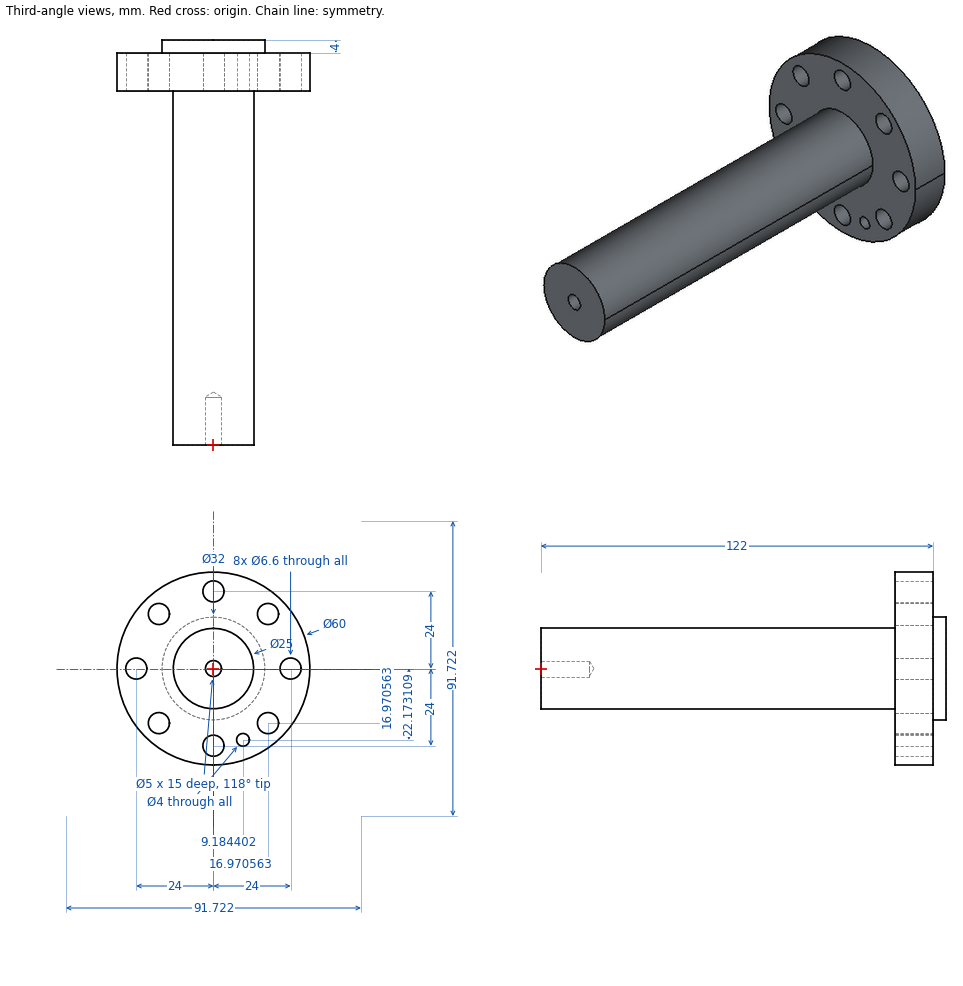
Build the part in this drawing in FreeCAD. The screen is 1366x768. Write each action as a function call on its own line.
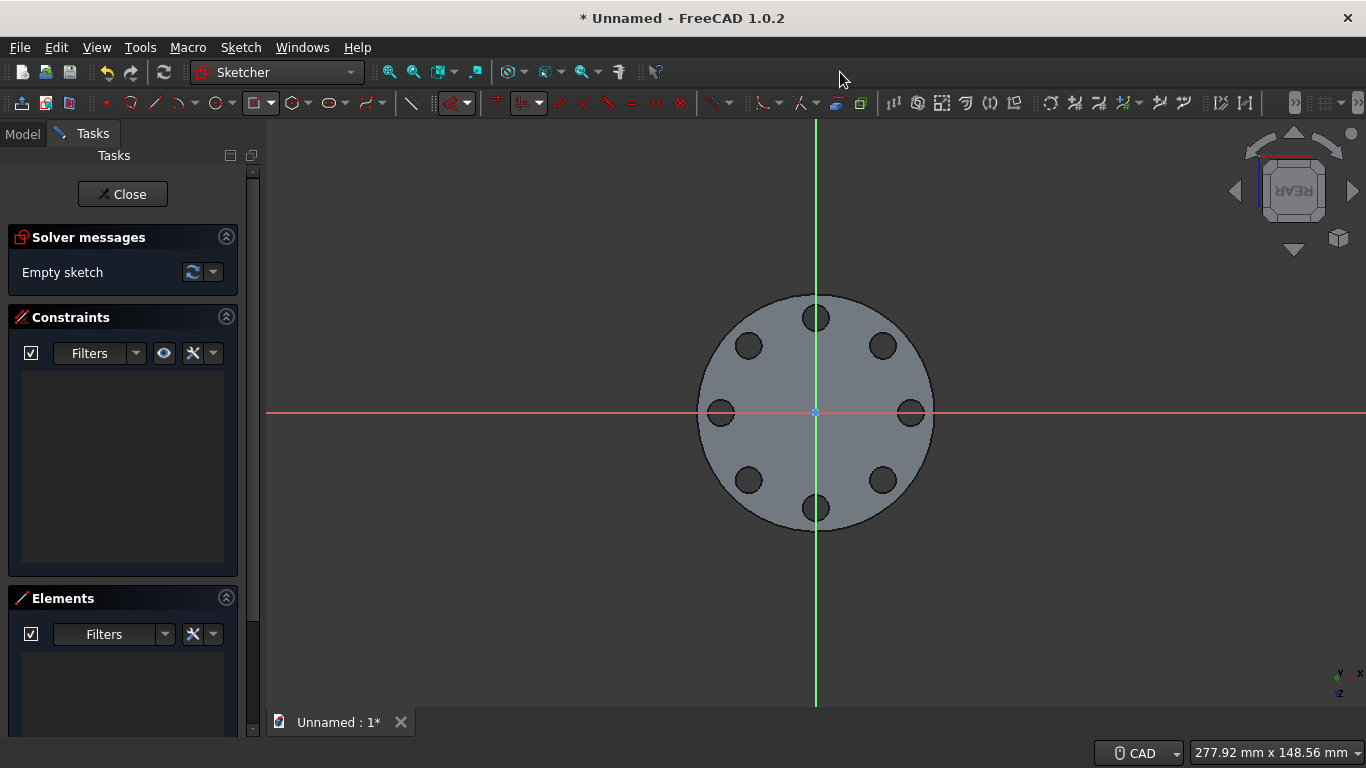
scroll(856, 413, up, 5)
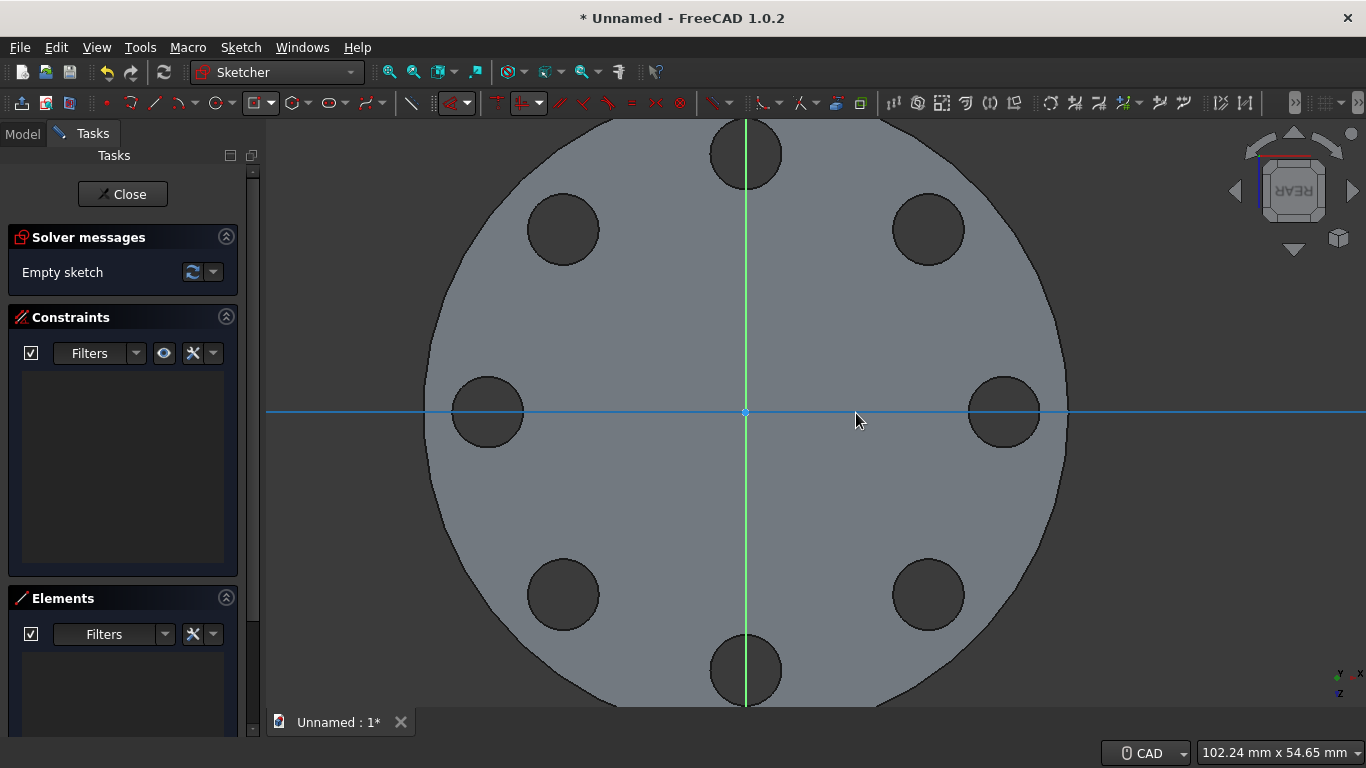
click(216, 104)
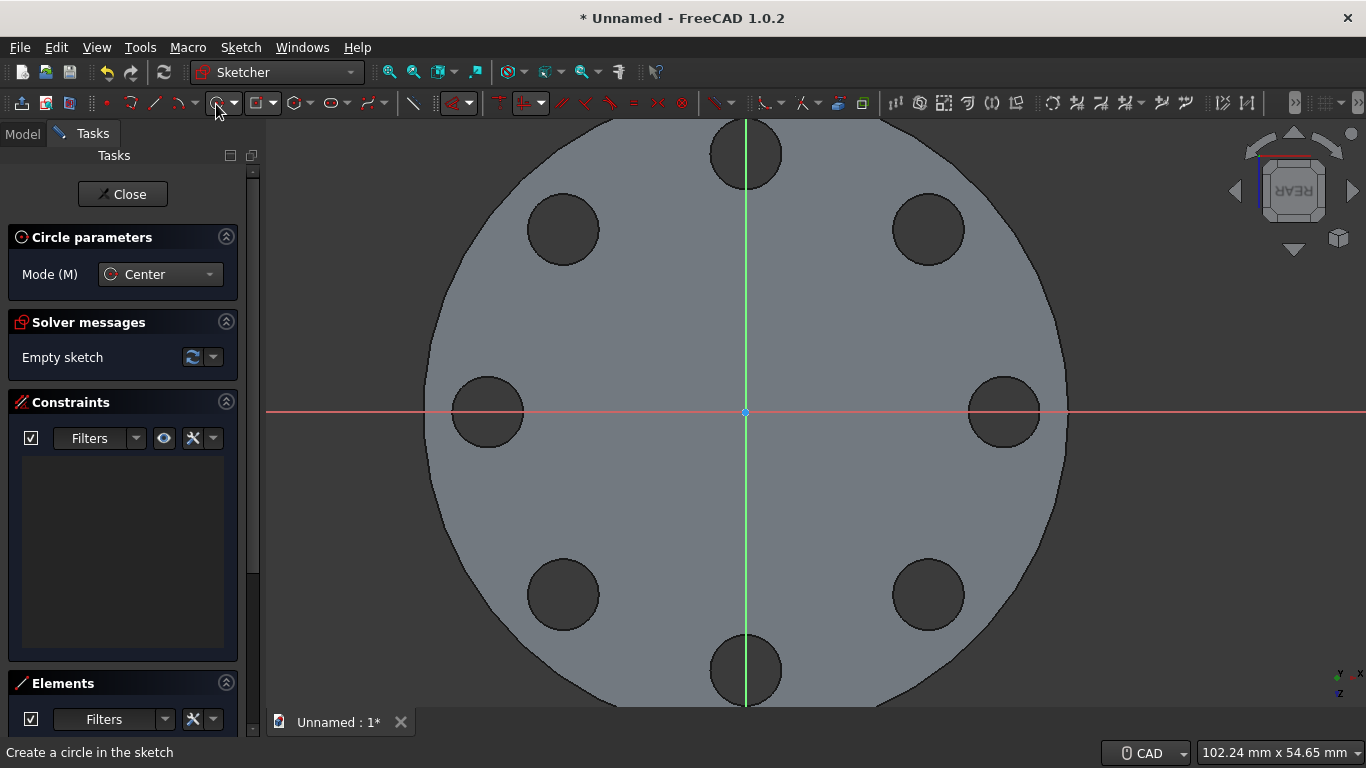
click(746, 412)
click(868, 290)
key(Escape)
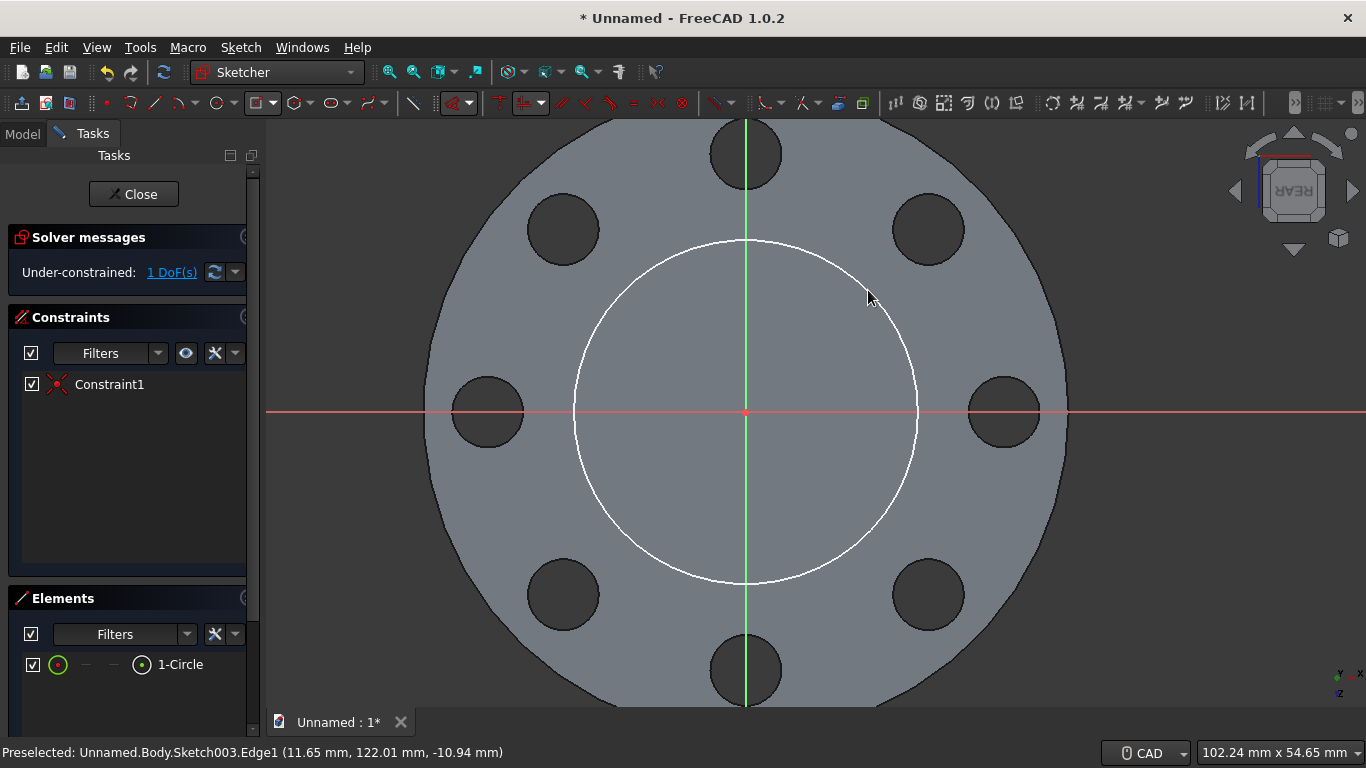
click(867, 290)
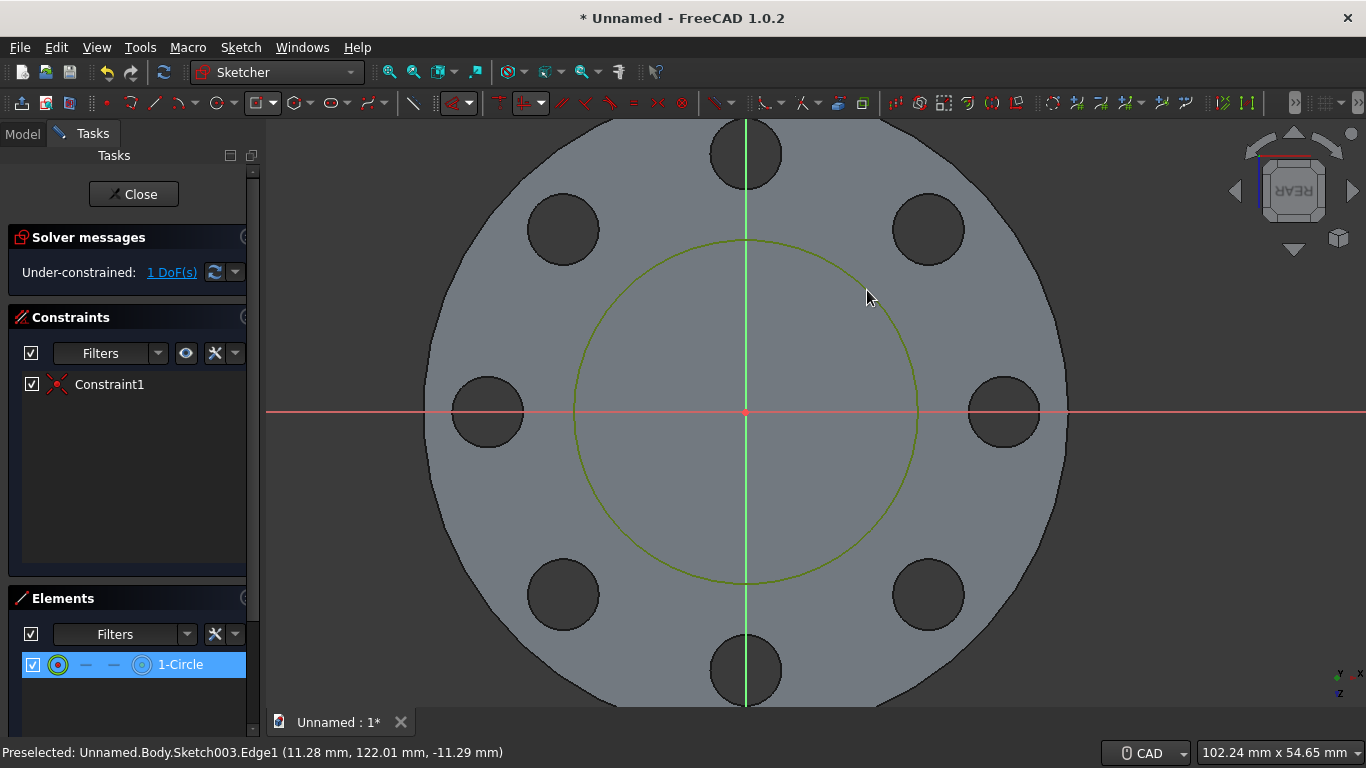
key(k)
key(o)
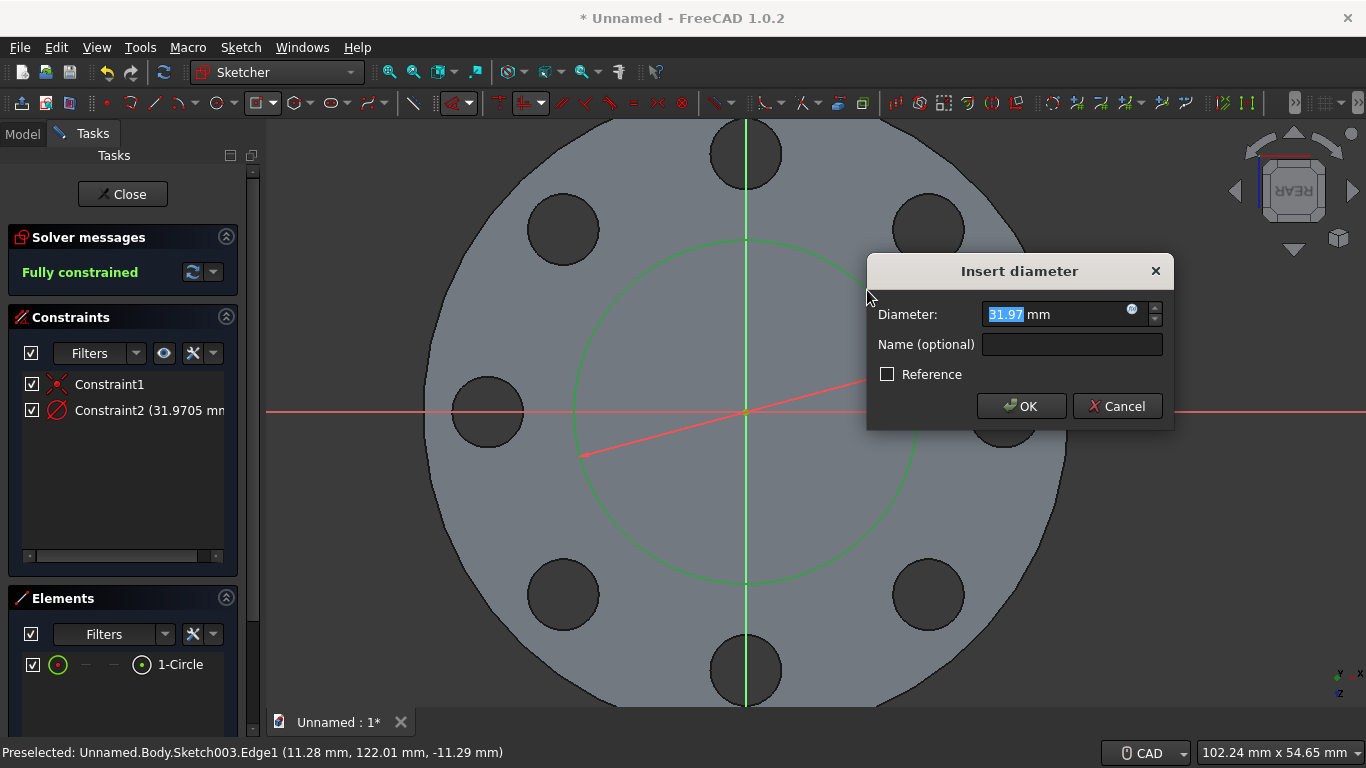
text(32)
key(Return)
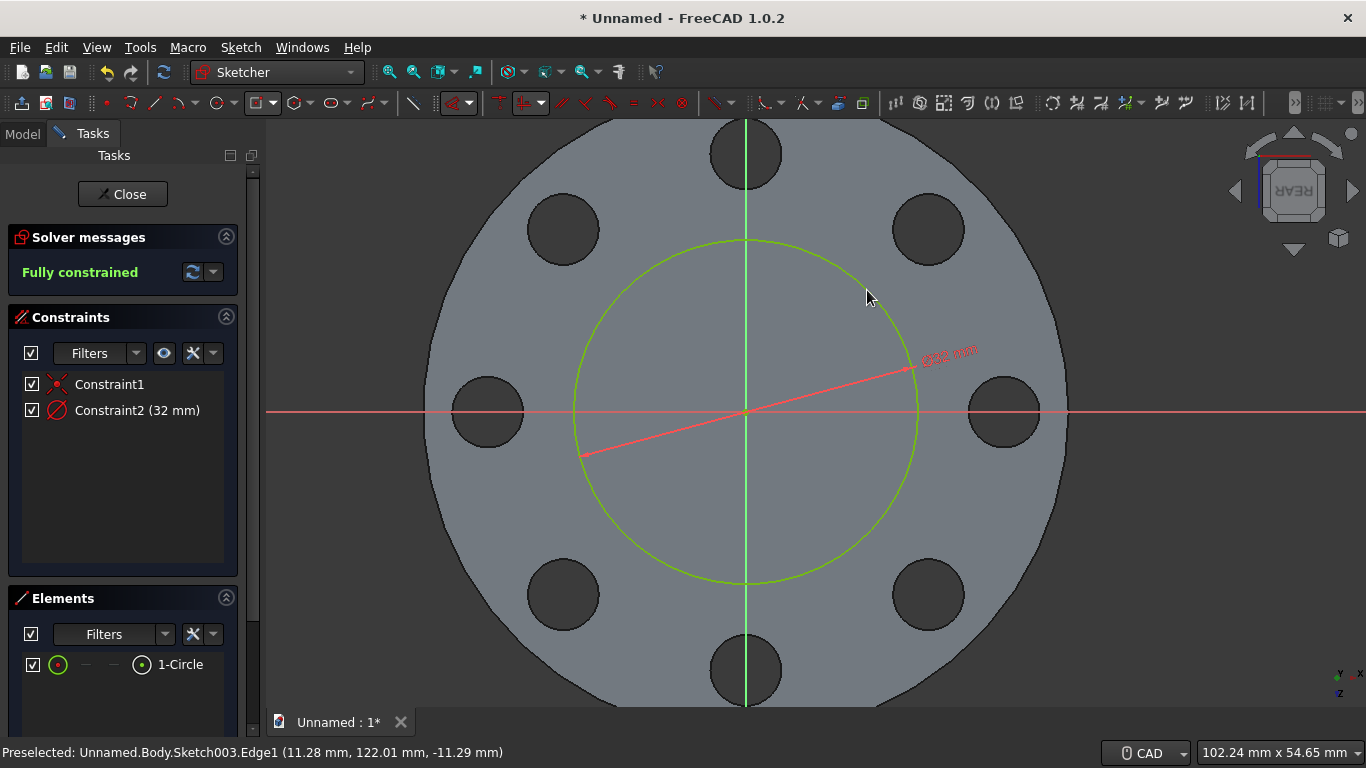
click(123, 194)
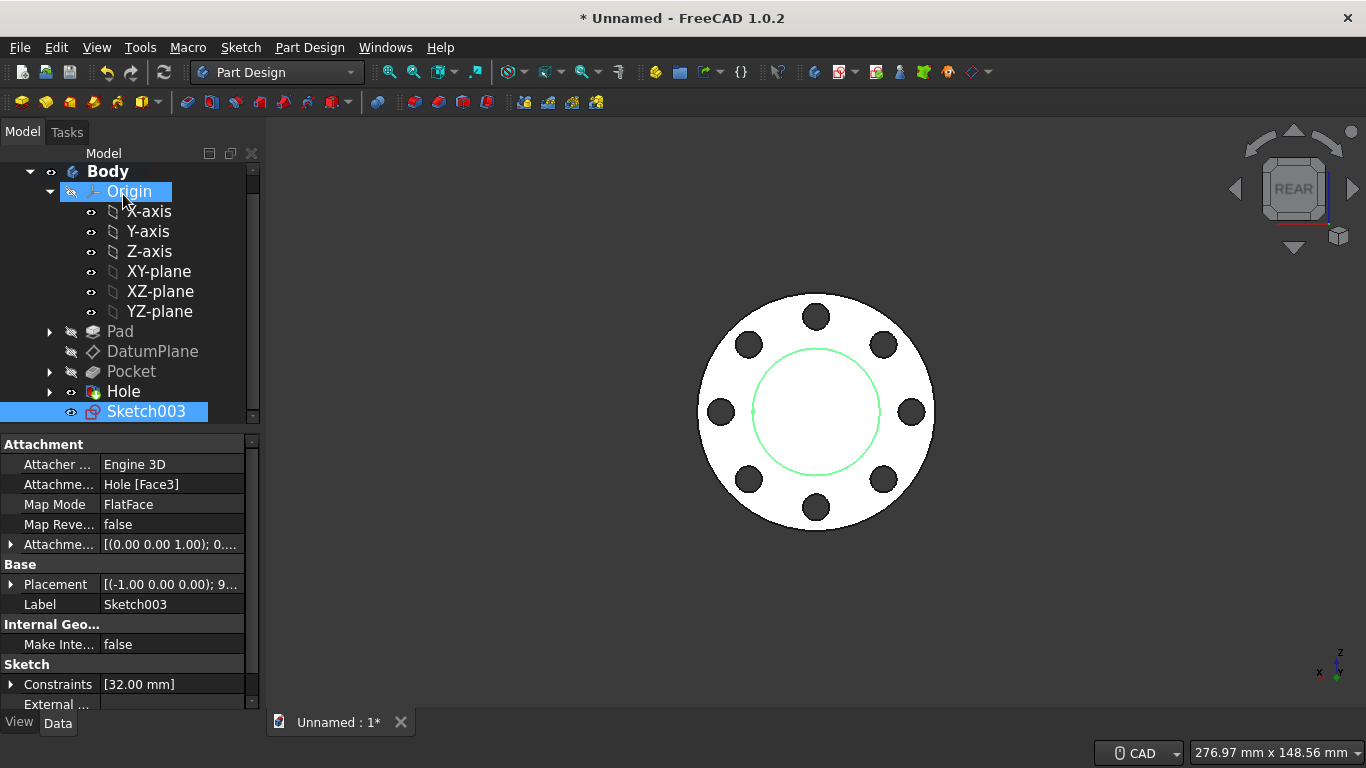
click(22, 102)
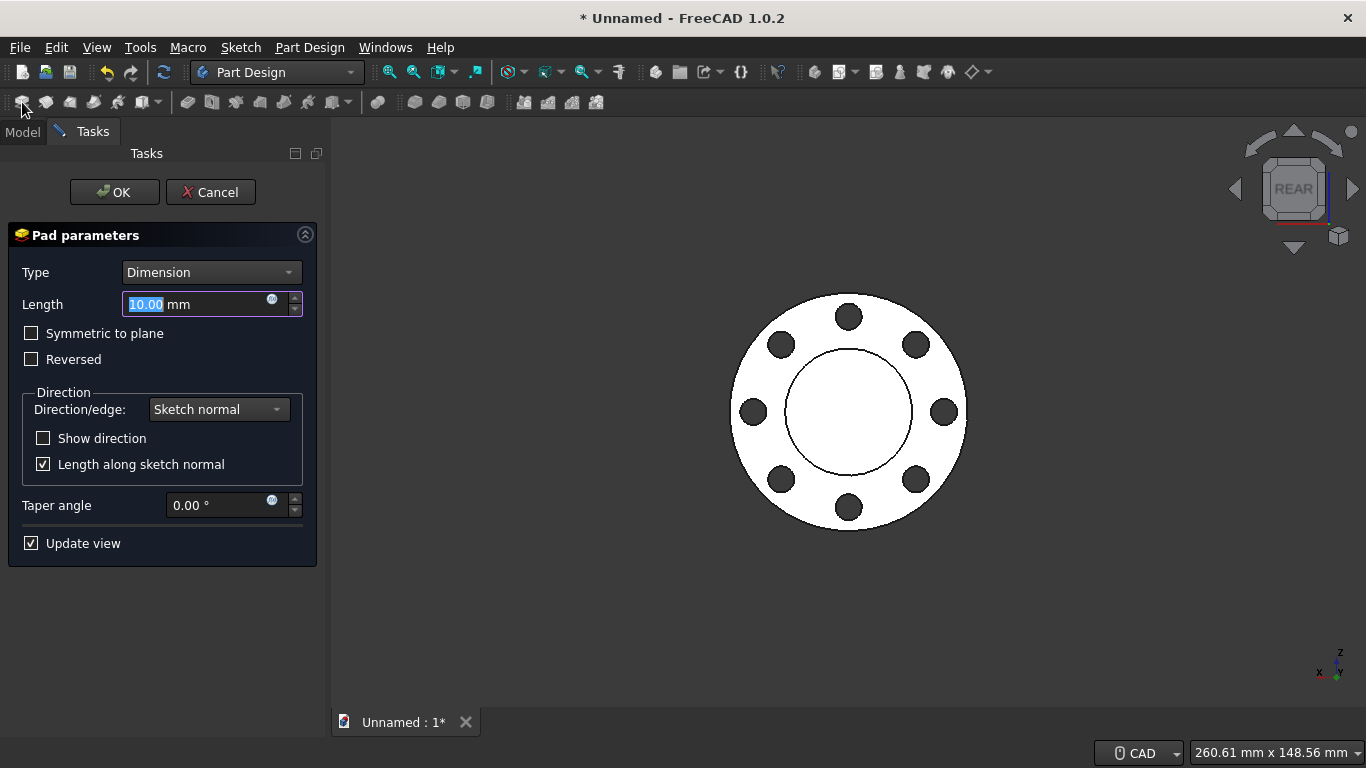
text(4)
key(Tab)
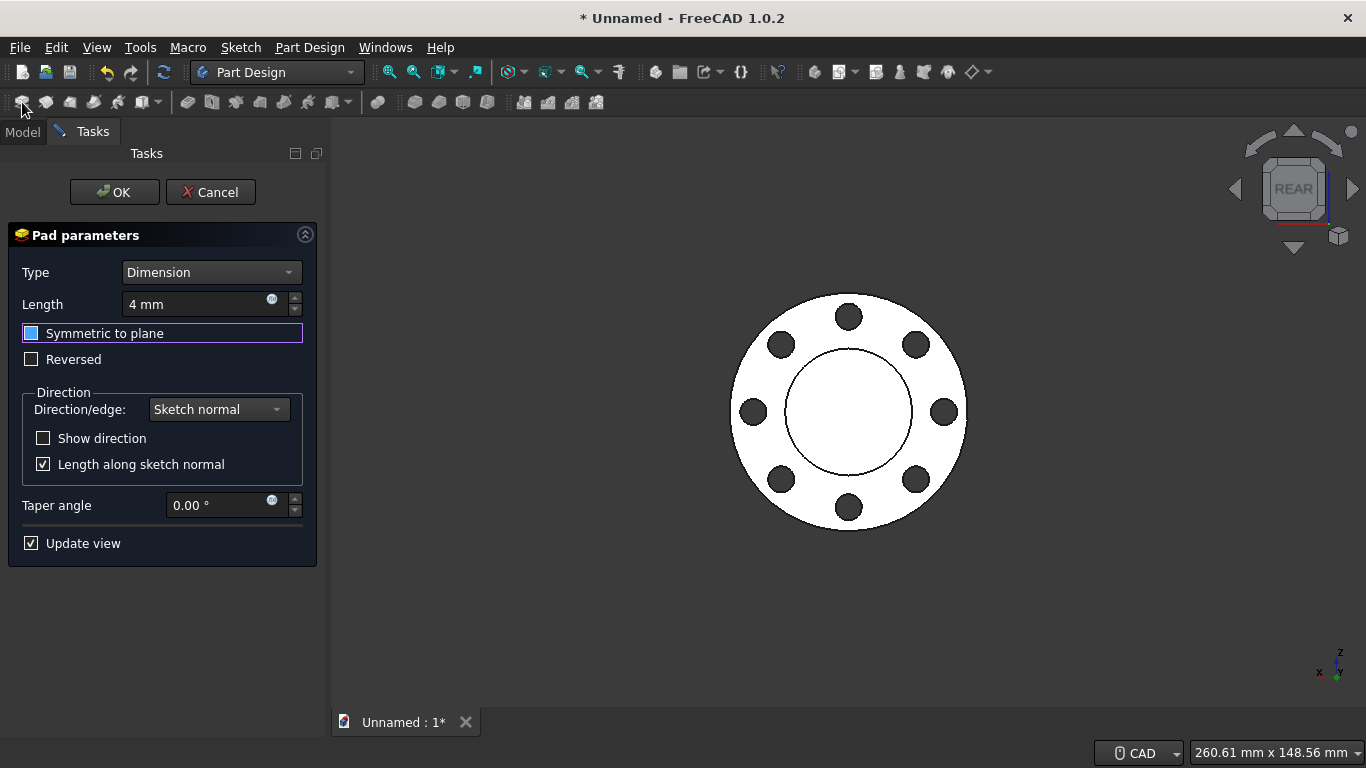
click(115, 192)